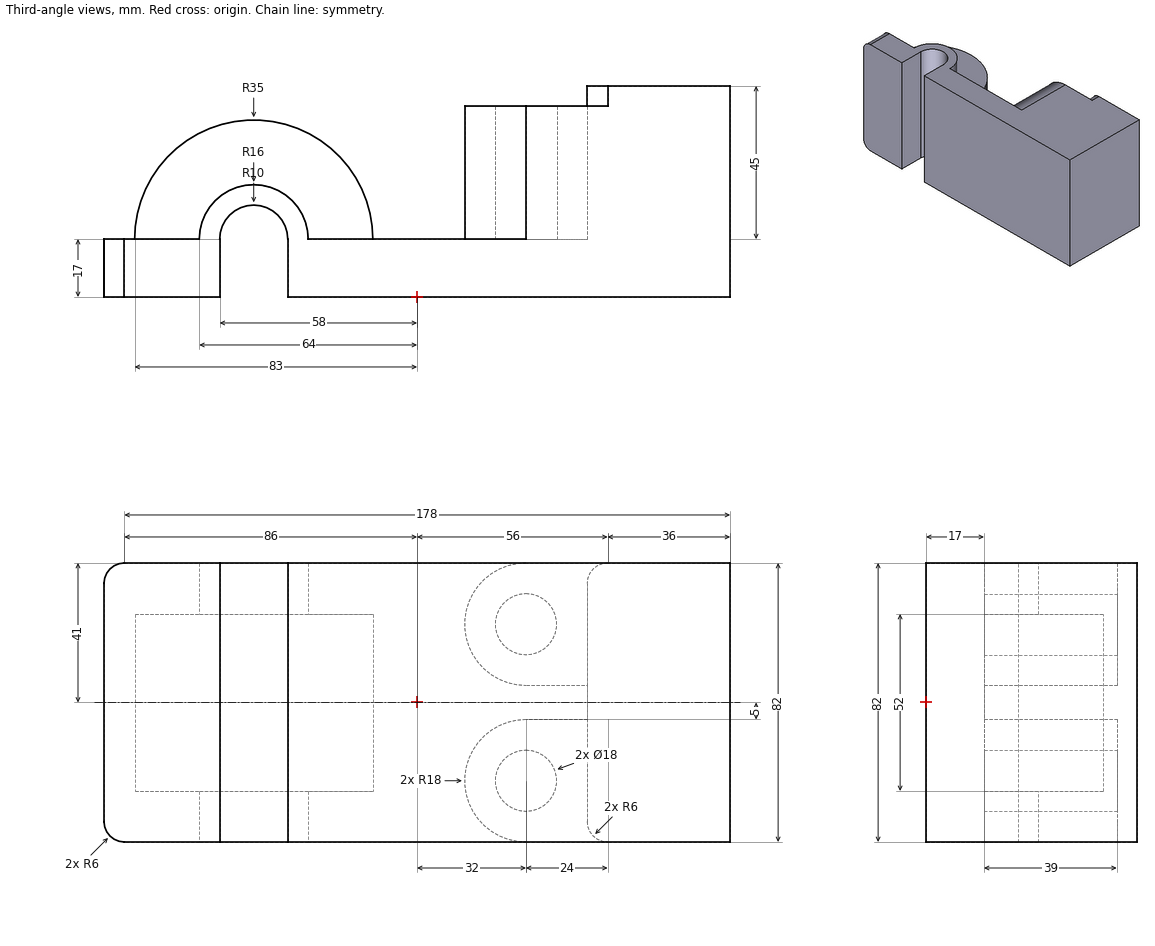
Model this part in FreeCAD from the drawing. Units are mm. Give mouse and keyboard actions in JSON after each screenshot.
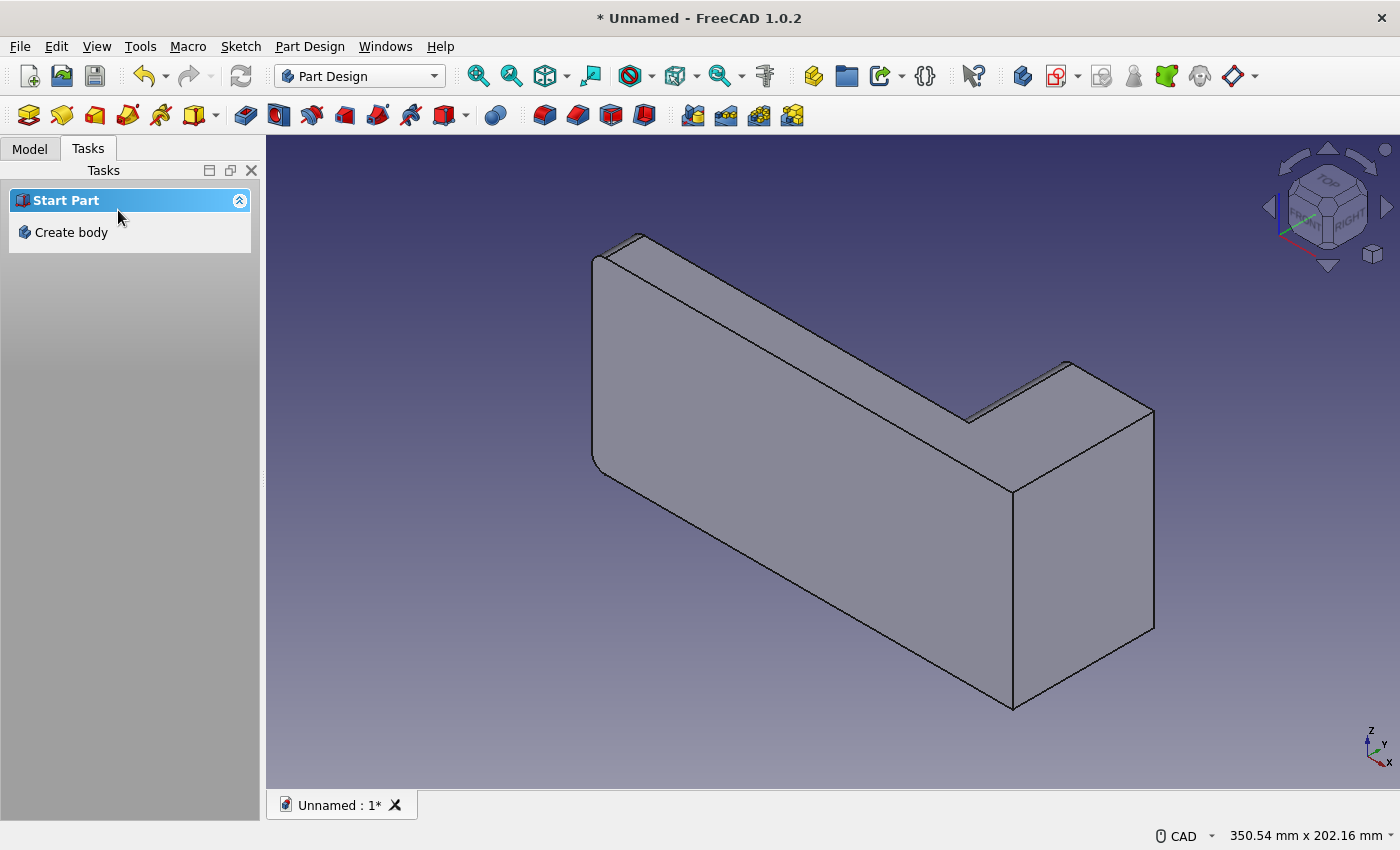
{"action": "left_click", "coordinate": [1095, 411]}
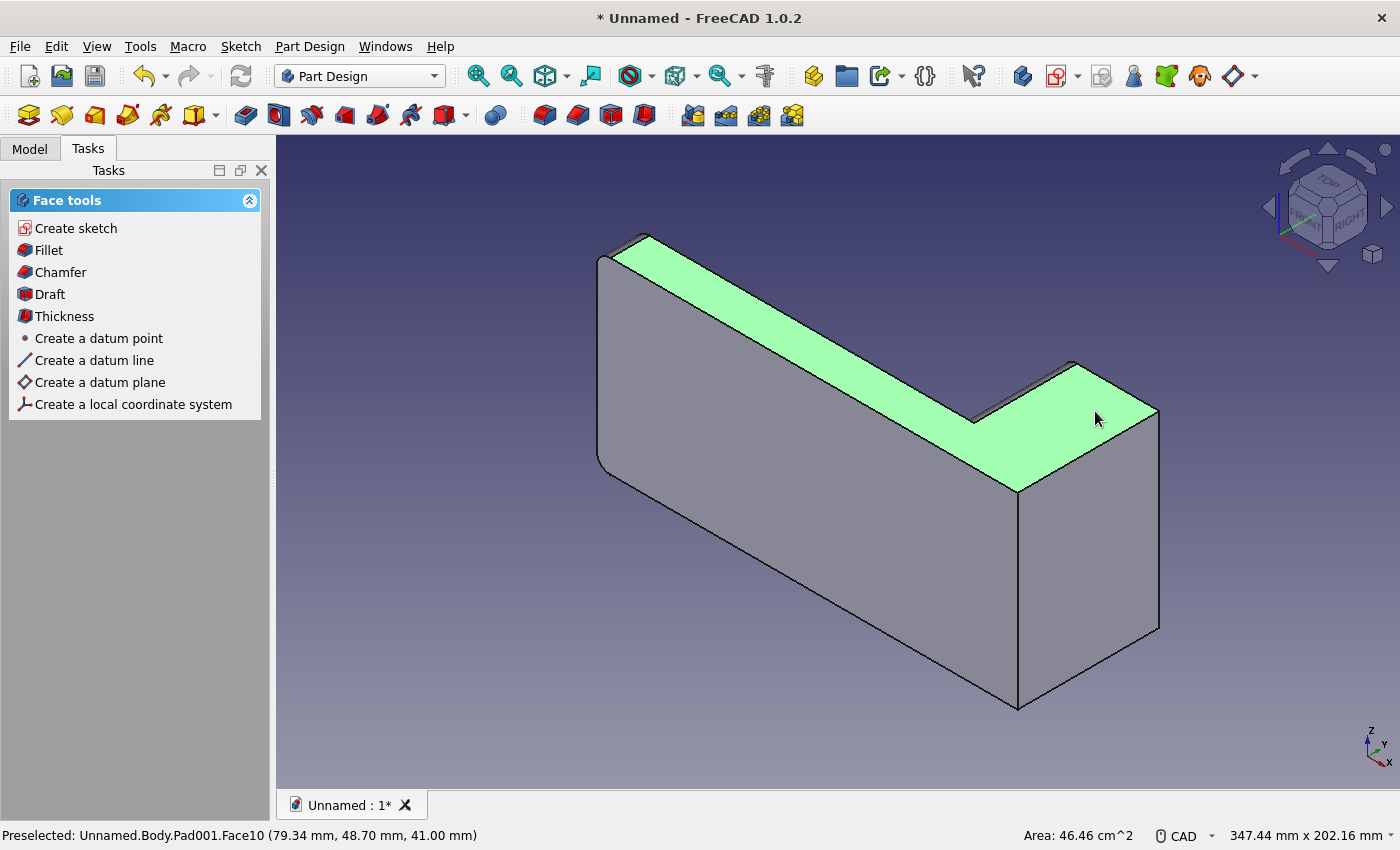
{"action": "left_click", "coordinate": [1056, 76]}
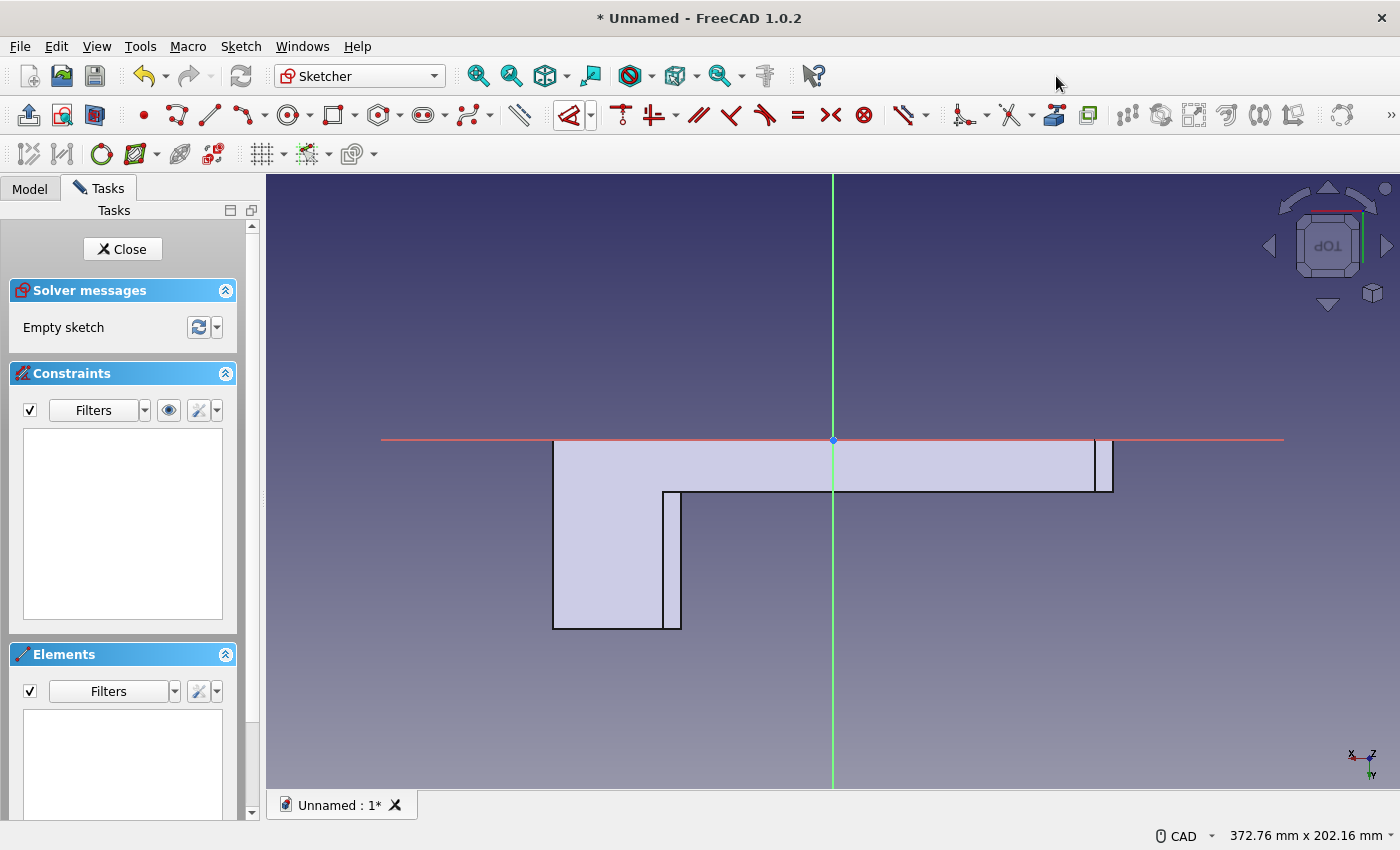
{"action": "scroll", "coordinate": [973, 482], "scroll_direction": "up", "scroll_amount": 7}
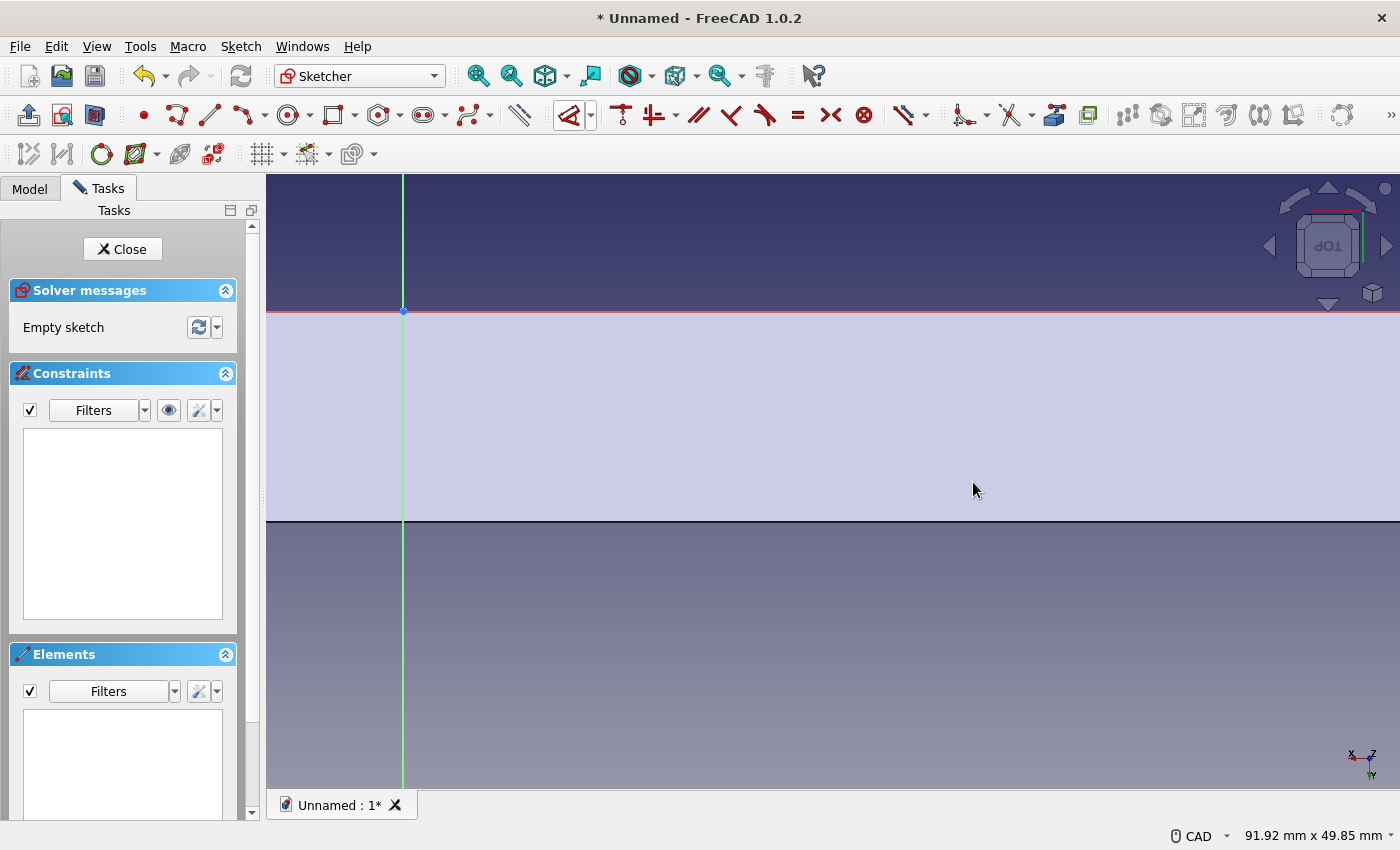
{"action": "left_click", "coordinate": [177, 116]}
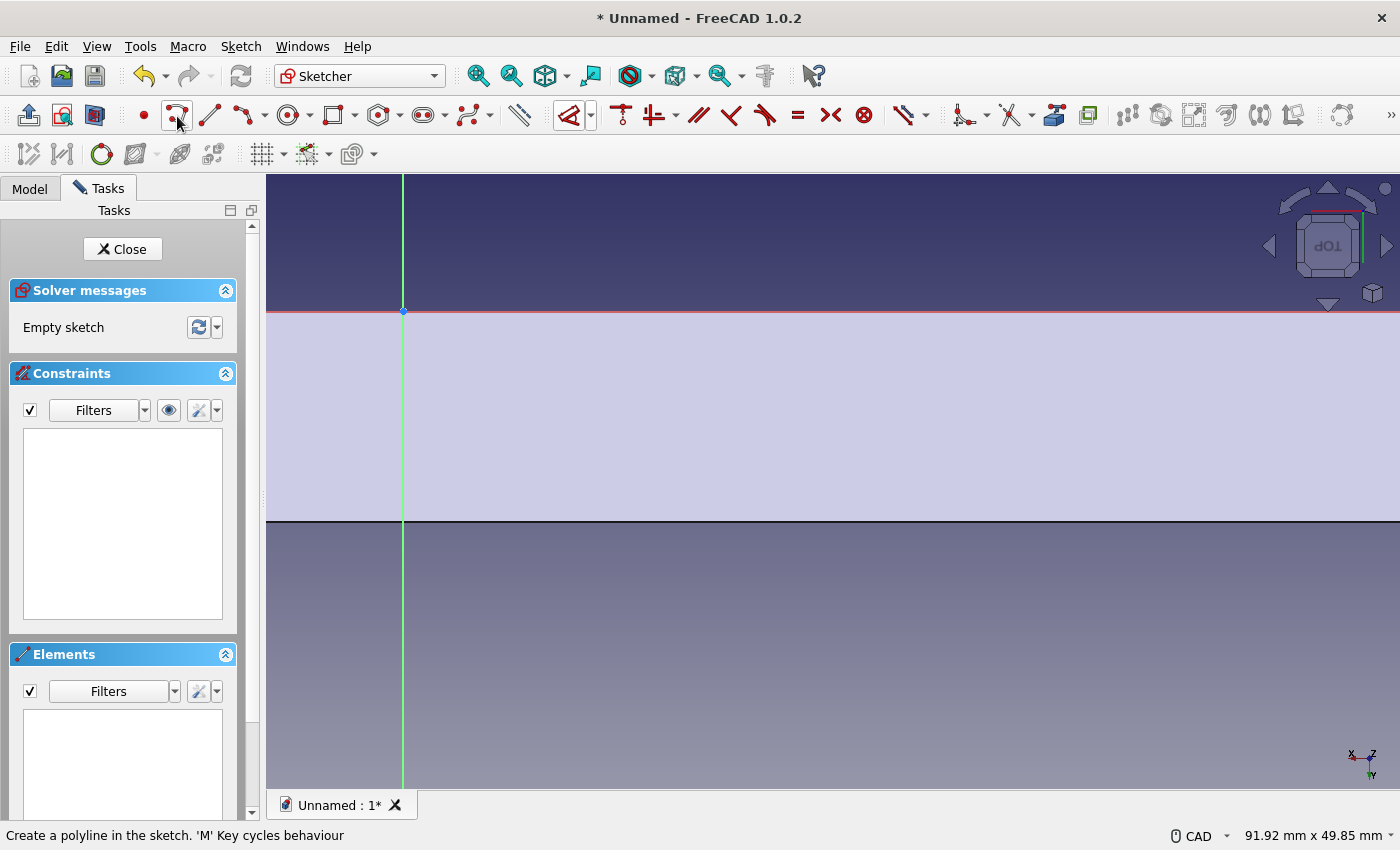
{"action": "left_click", "coordinate": [1119, 522]}
{"action": "left_click", "coordinate": [1119, 312]}
{"action": "left_click", "coordinate": [872, 321]}
{"action": "left_click", "coordinate": [872, 522]}
{"action": "right_click", "coordinate": [872, 522]}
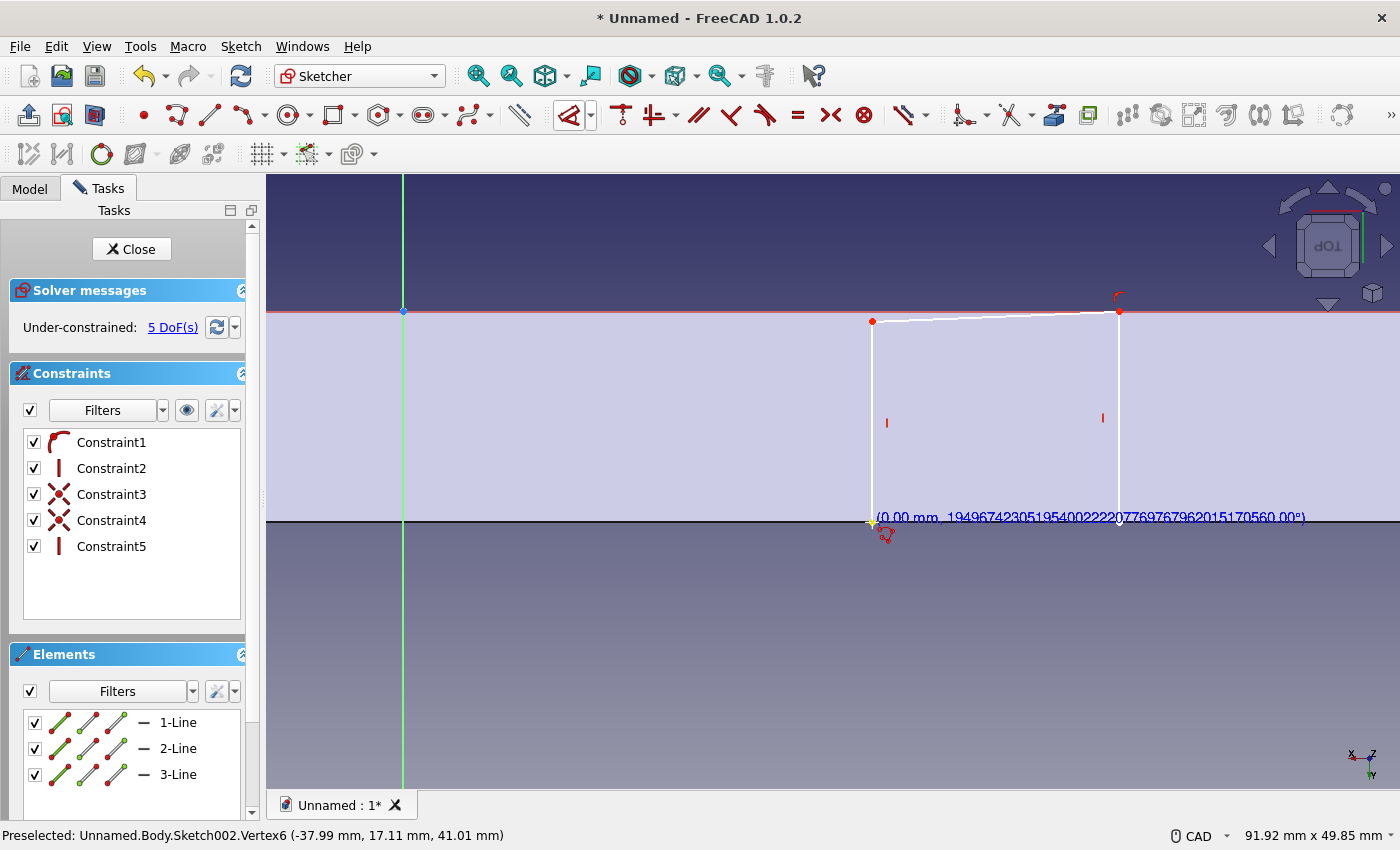
{"action": "left_click", "coordinate": [242, 116]}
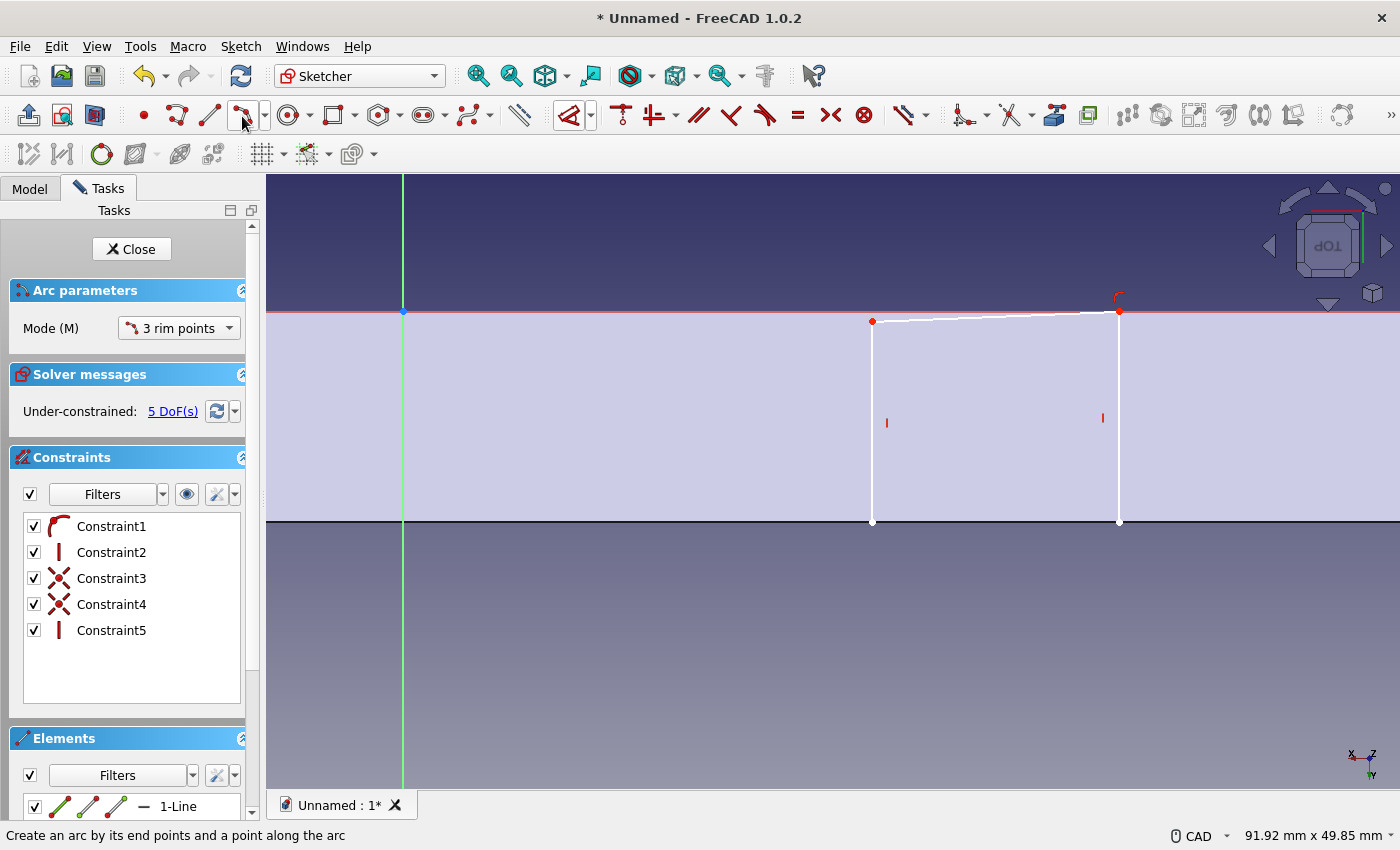
{"action": "left_click", "coordinate": [872, 523]}
{"action": "left_click", "coordinate": [1119, 523]}
{"action": "left_click", "coordinate": [996, 645]}
{"action": "key", "text": "Escape"}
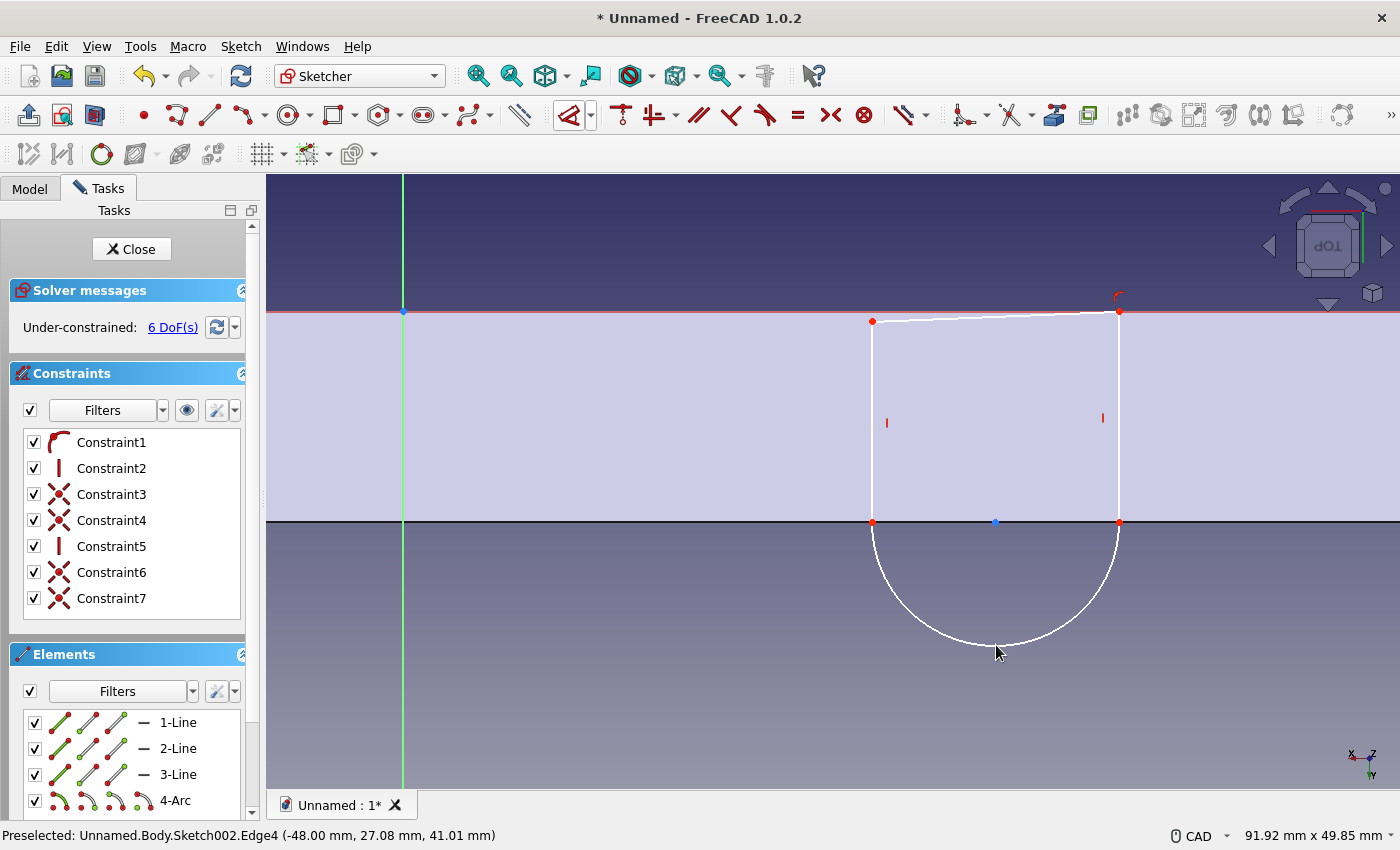
{"action": "left_click", "coordinate": [1119, 460]}